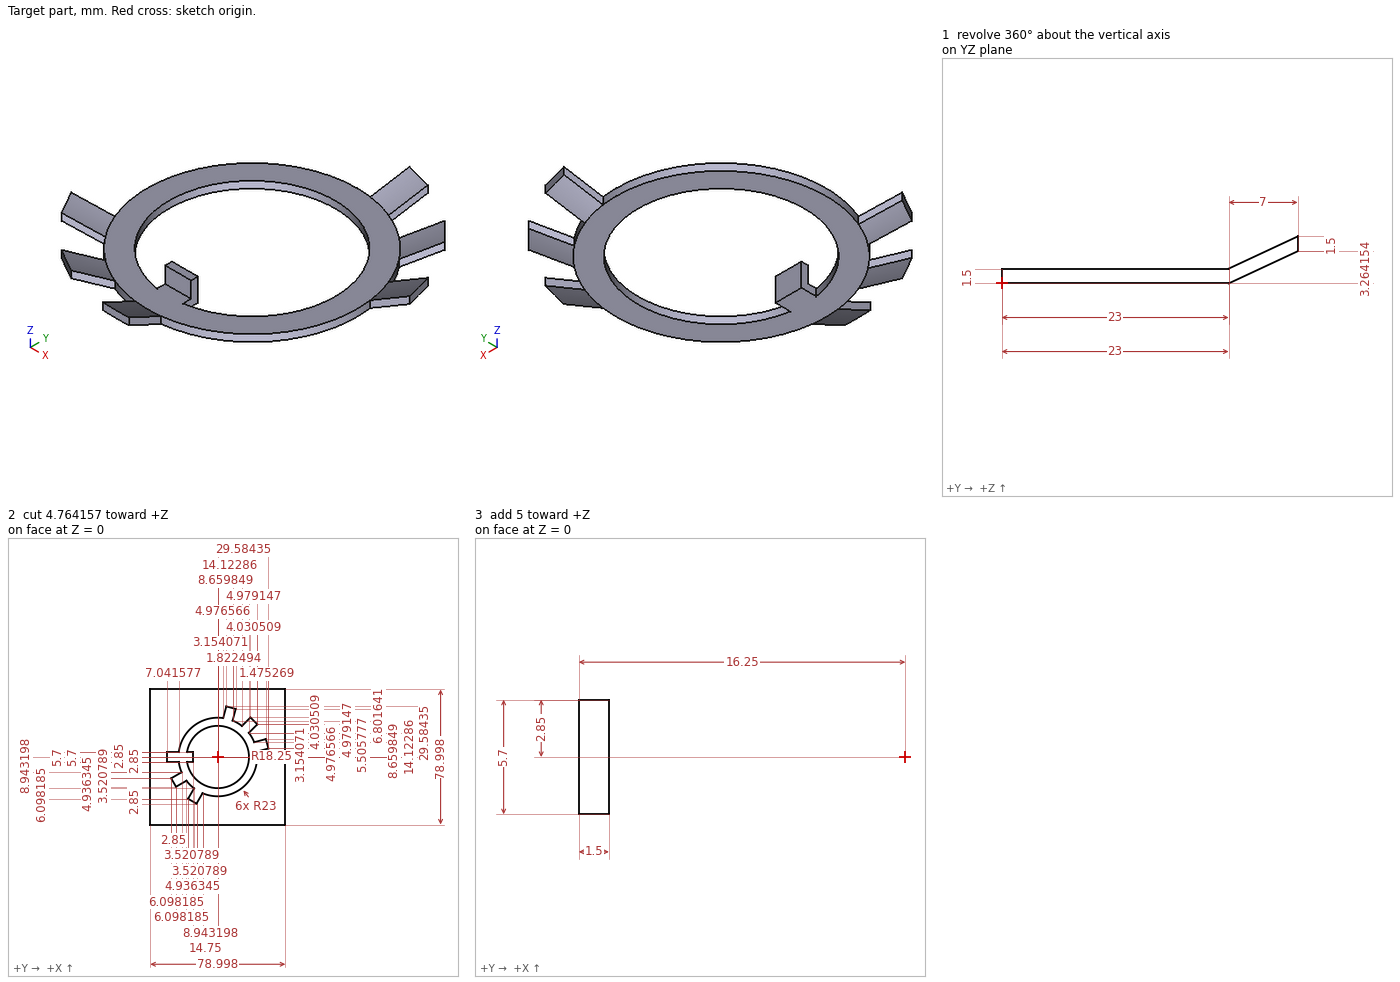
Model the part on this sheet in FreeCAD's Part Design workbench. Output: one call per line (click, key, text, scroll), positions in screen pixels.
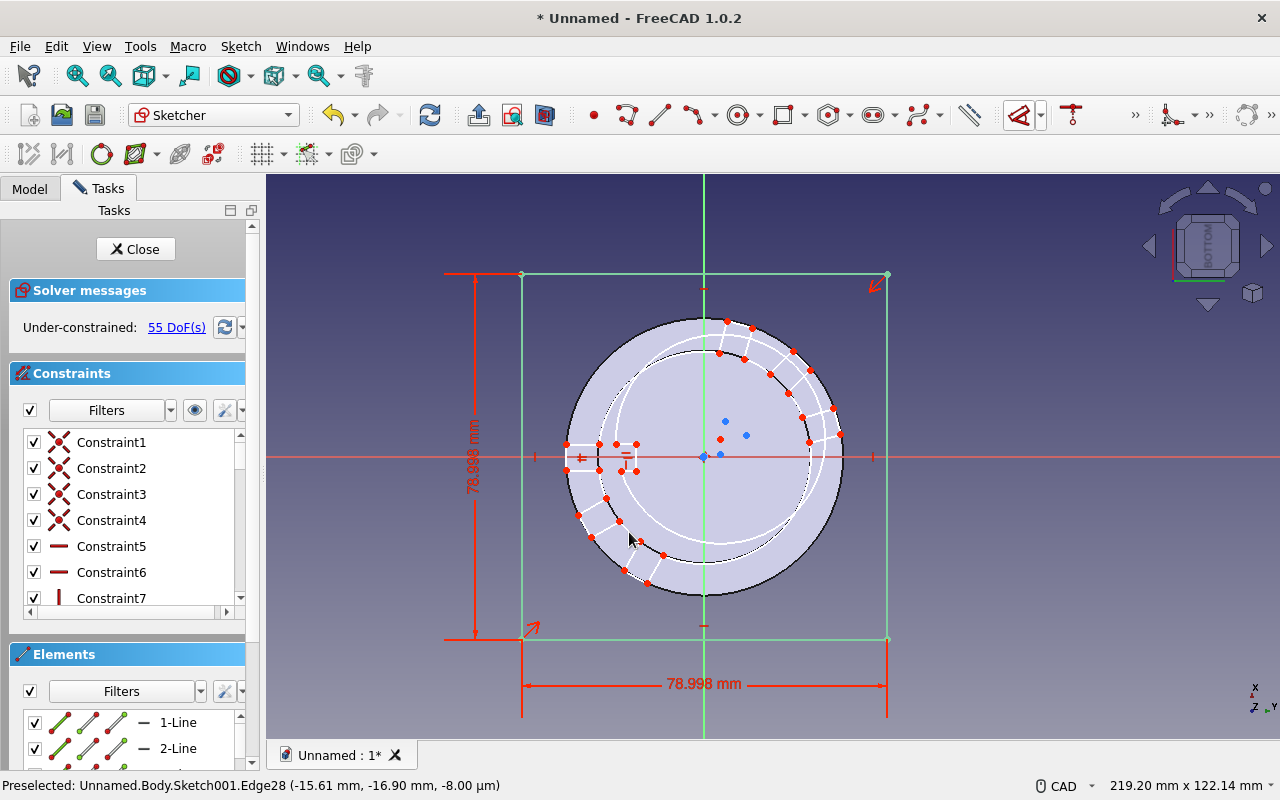
scroll(740, 336, up, 2)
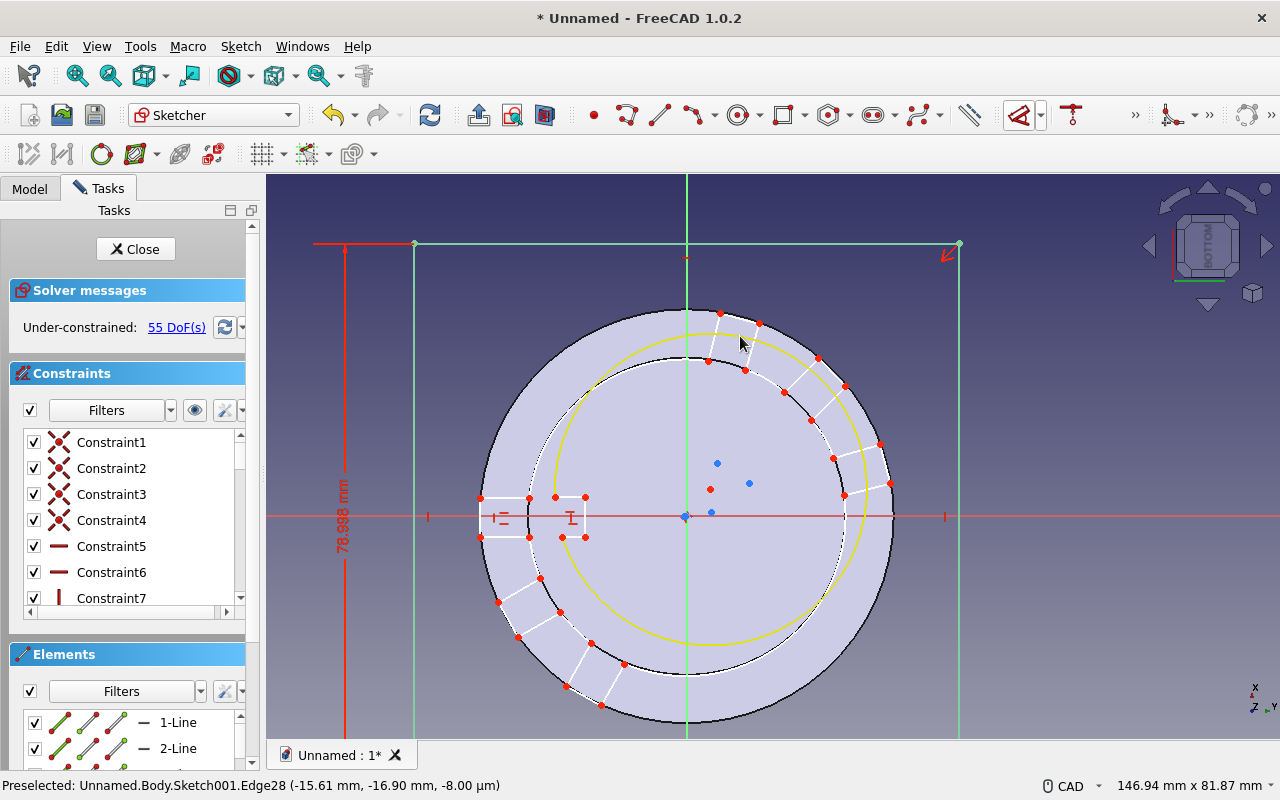
click(740, 336)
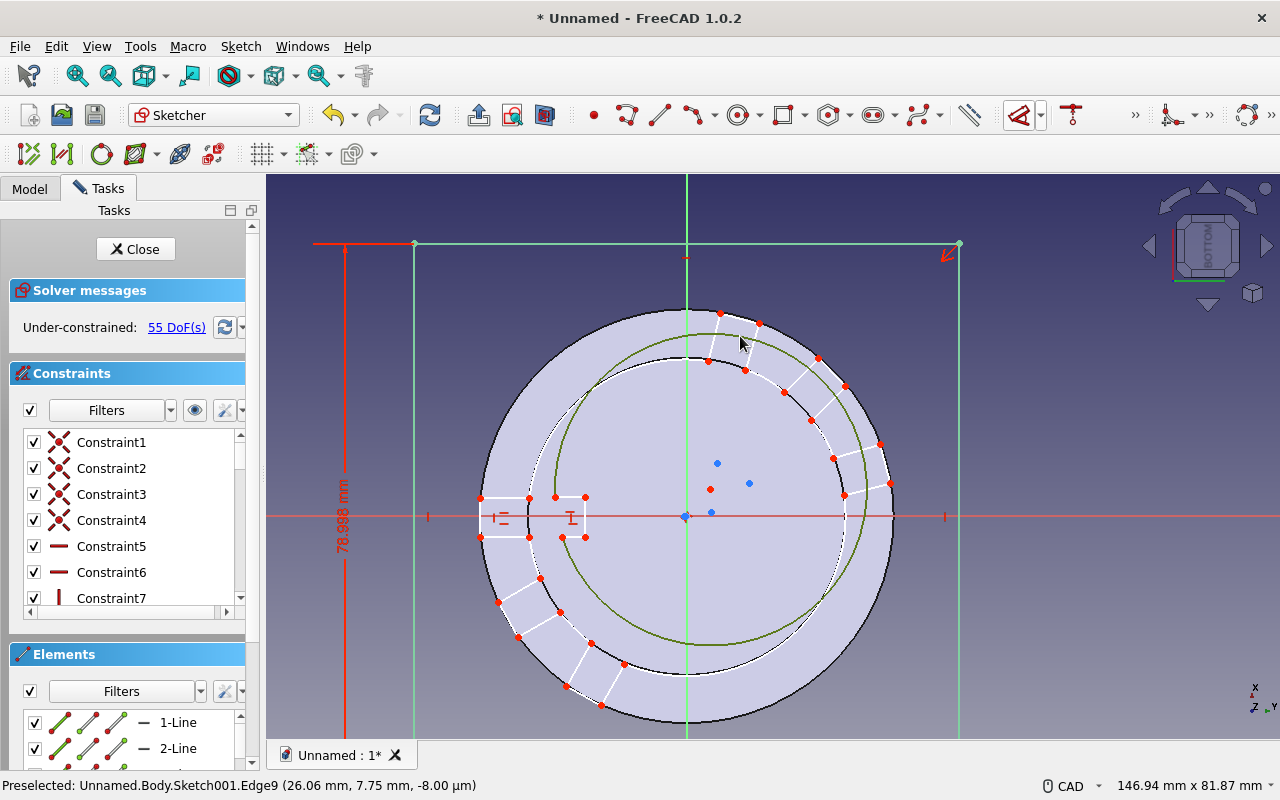
click(723, 672)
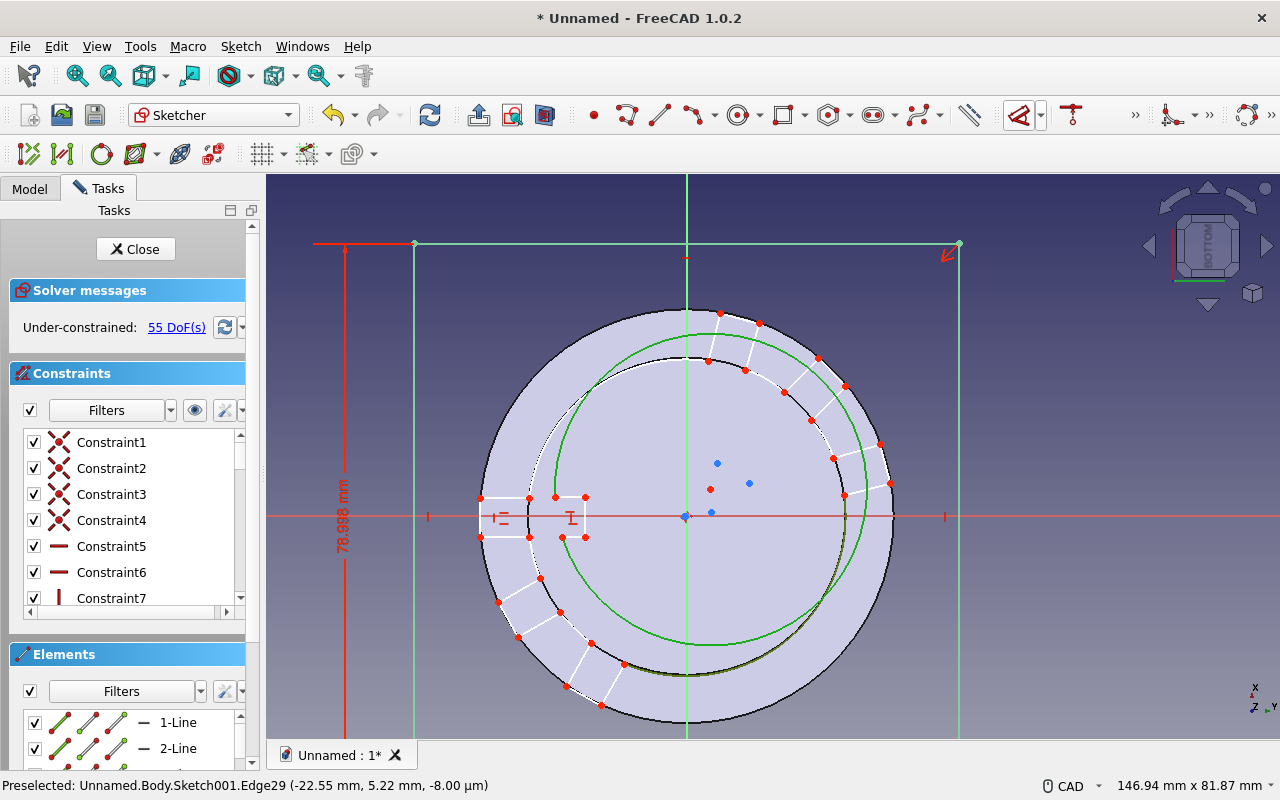
click(1071, 116)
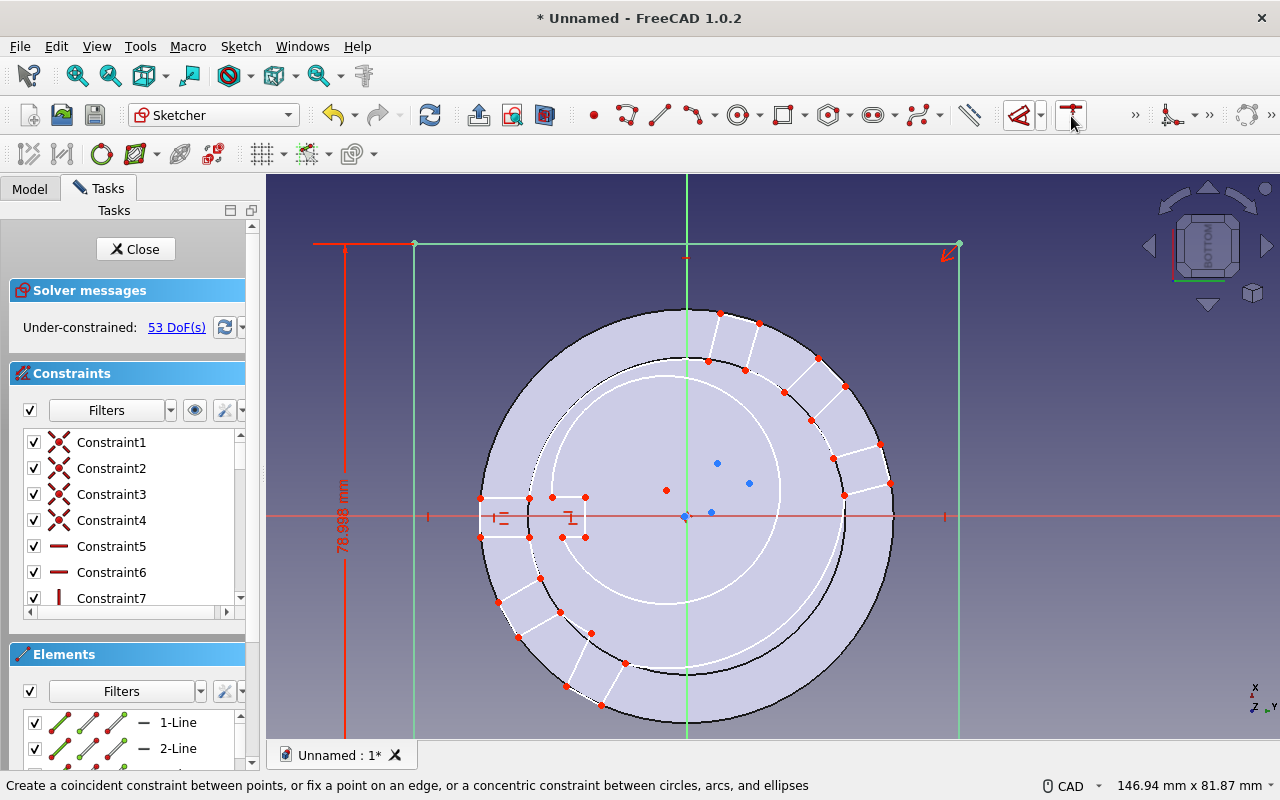
click(734, 582)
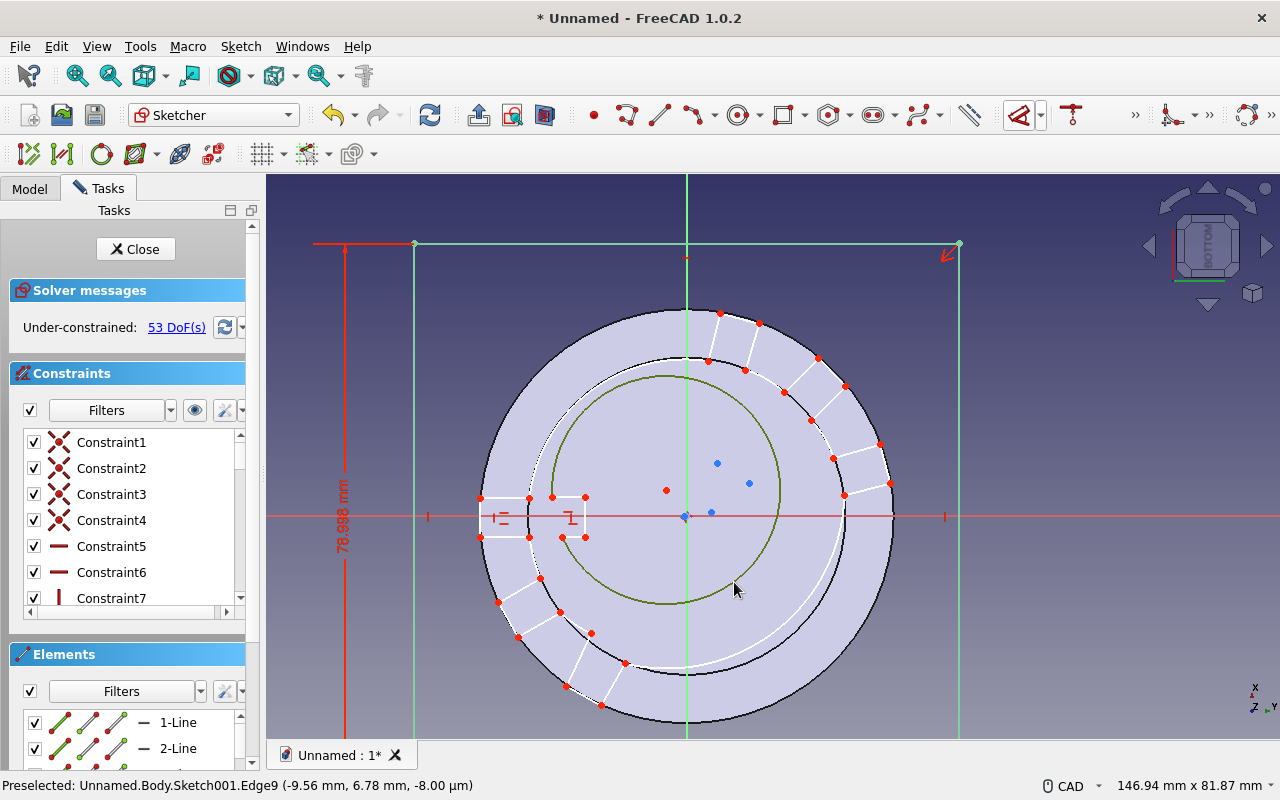
click(829, 446)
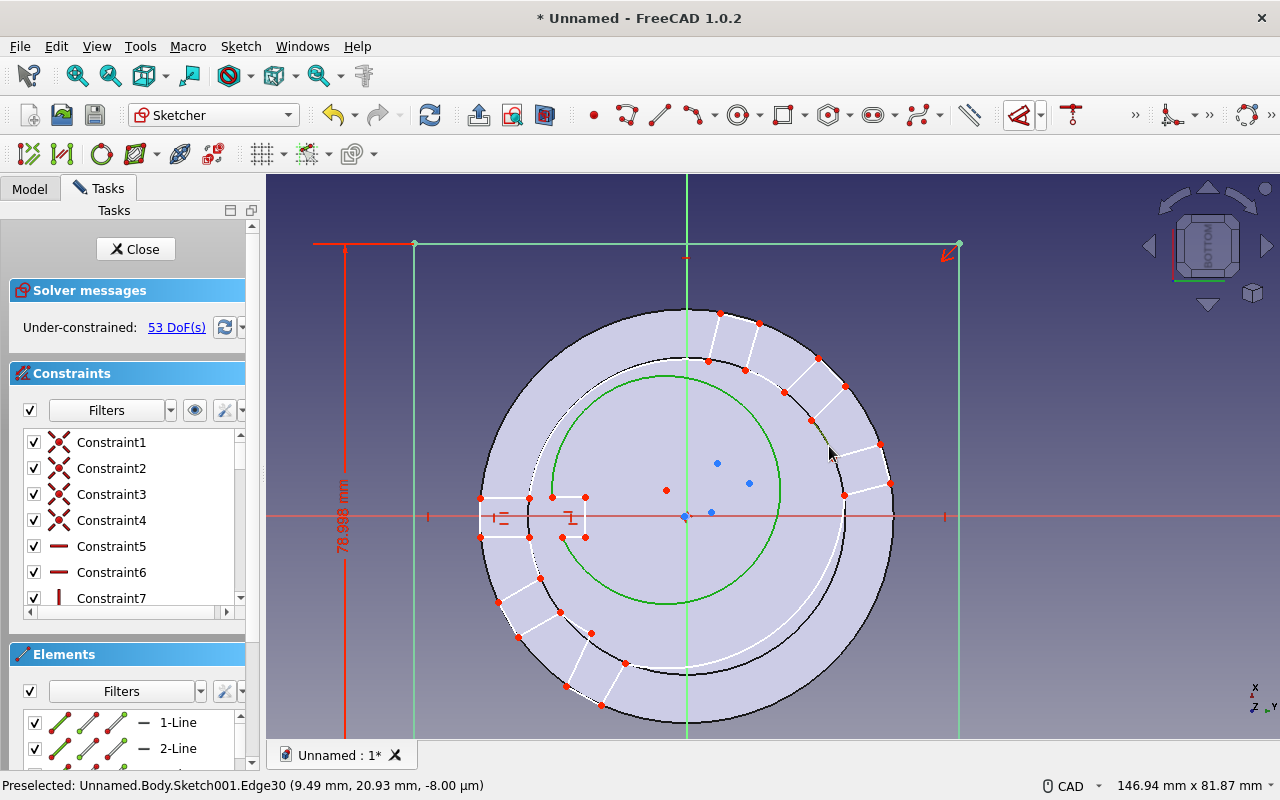
click(1071, 116)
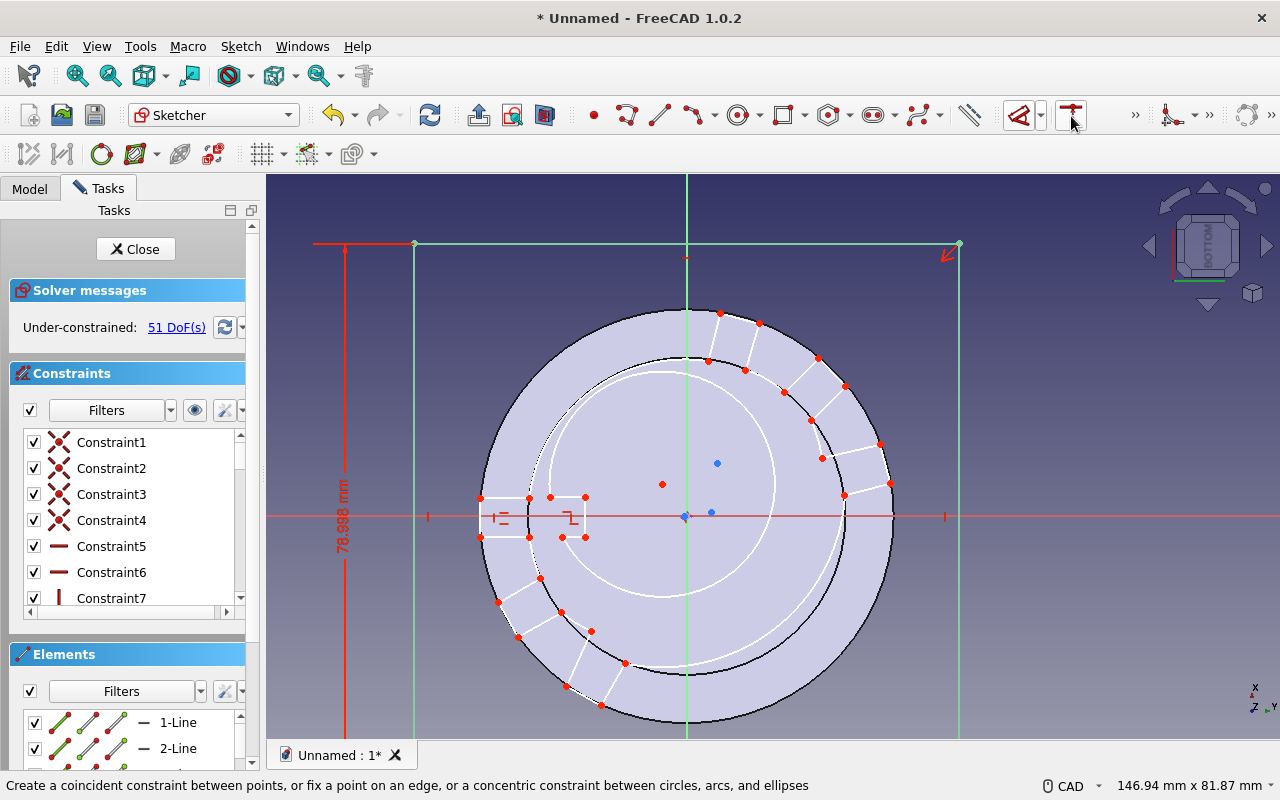
click(734, 571)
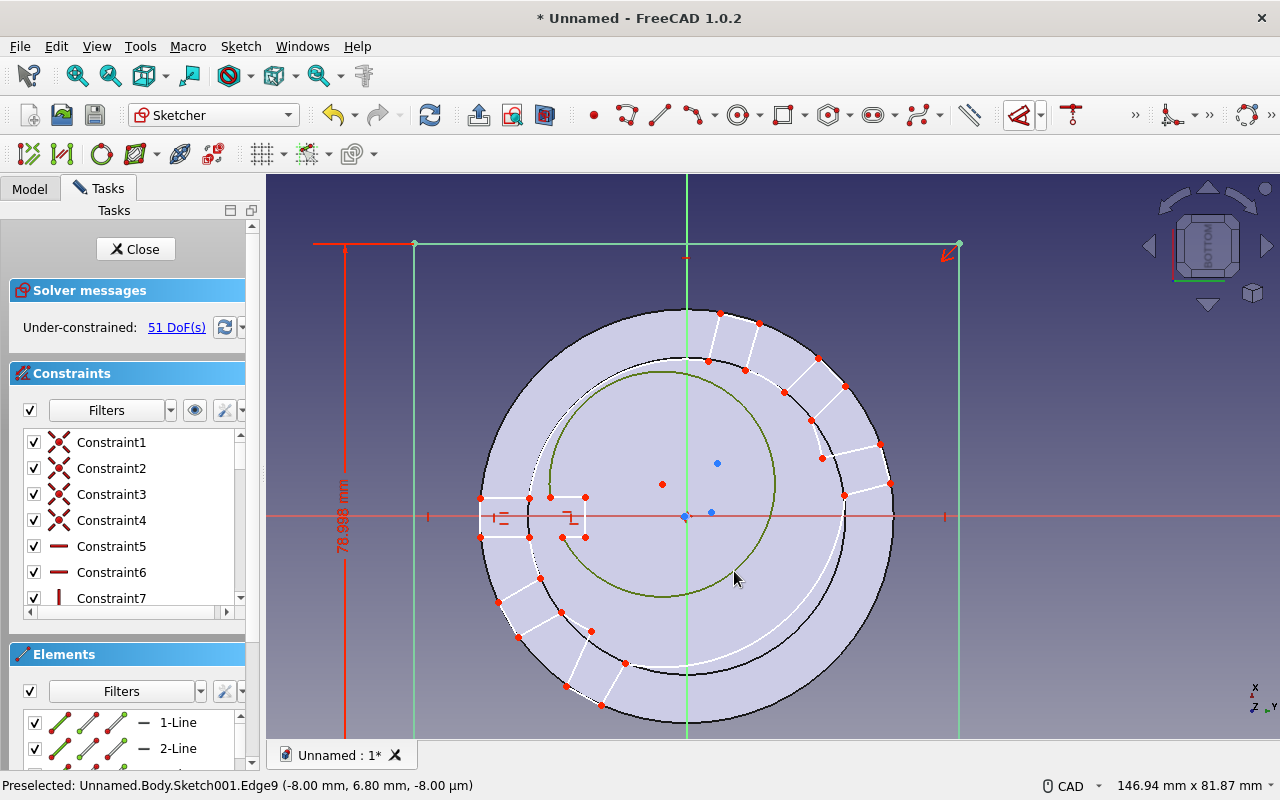
click(774, 384)